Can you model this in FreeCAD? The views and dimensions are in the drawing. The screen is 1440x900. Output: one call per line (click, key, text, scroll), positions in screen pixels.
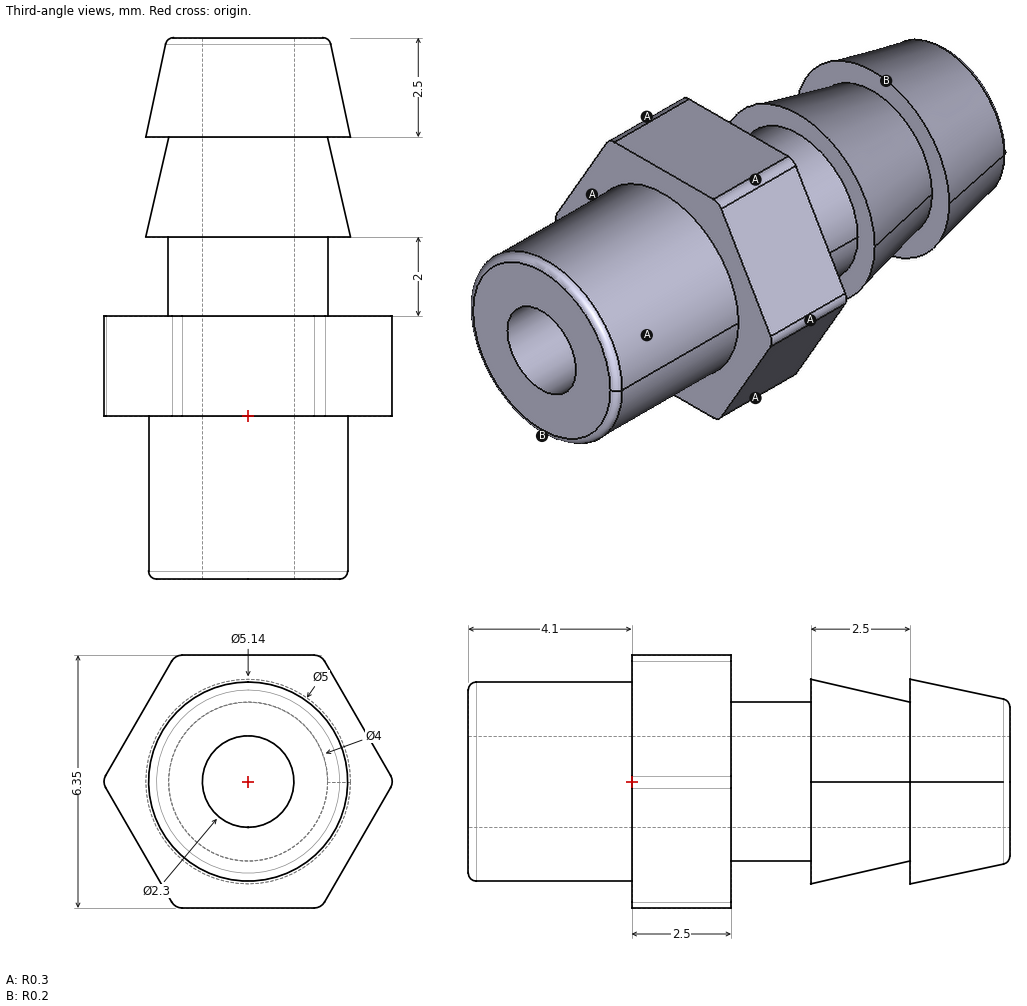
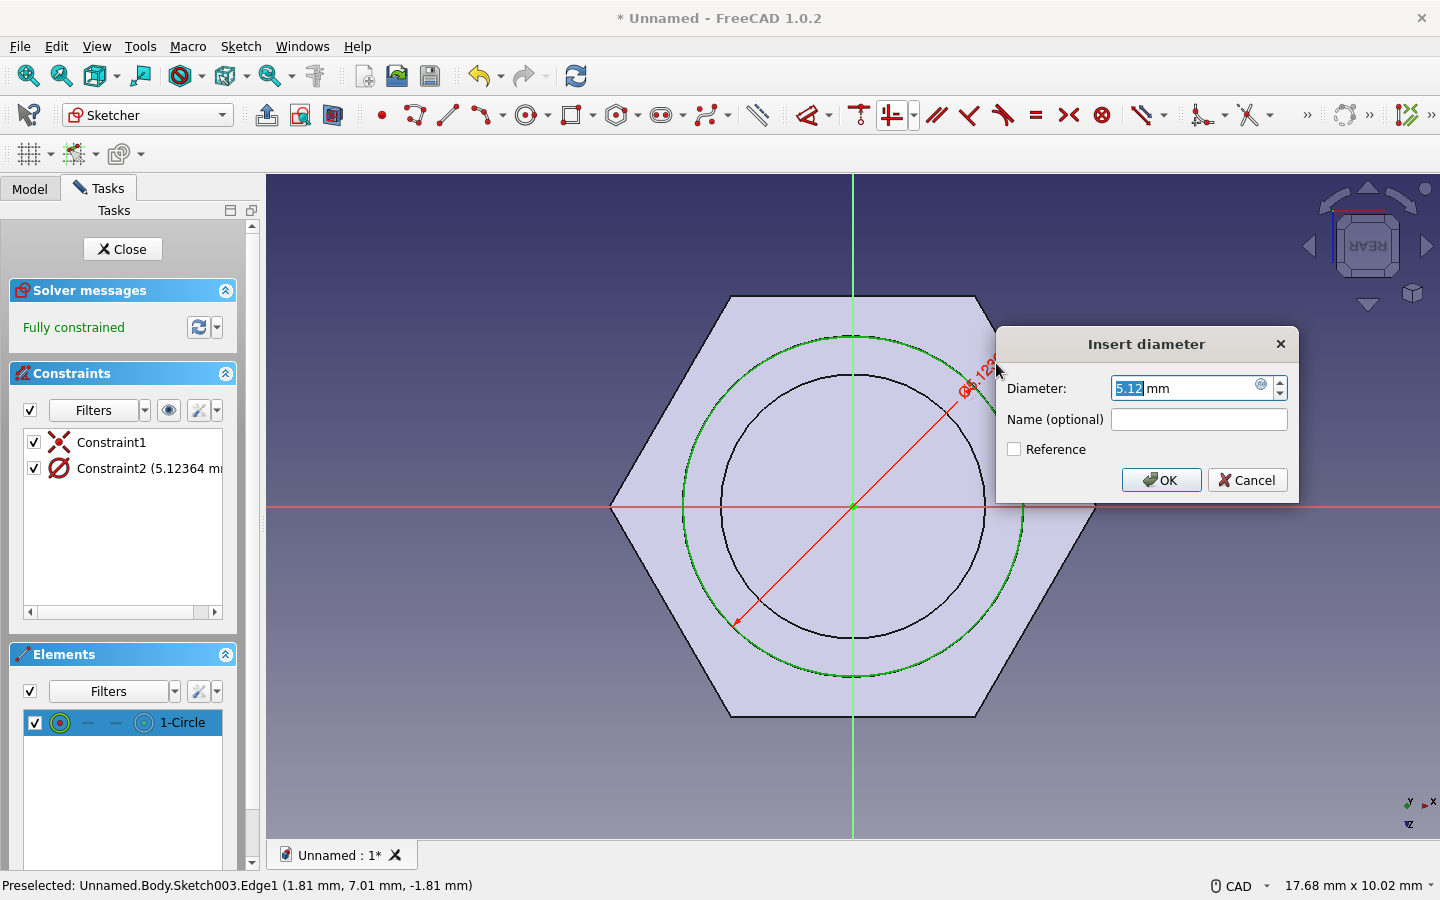
text(5.14)
key(Return)
key(Escape)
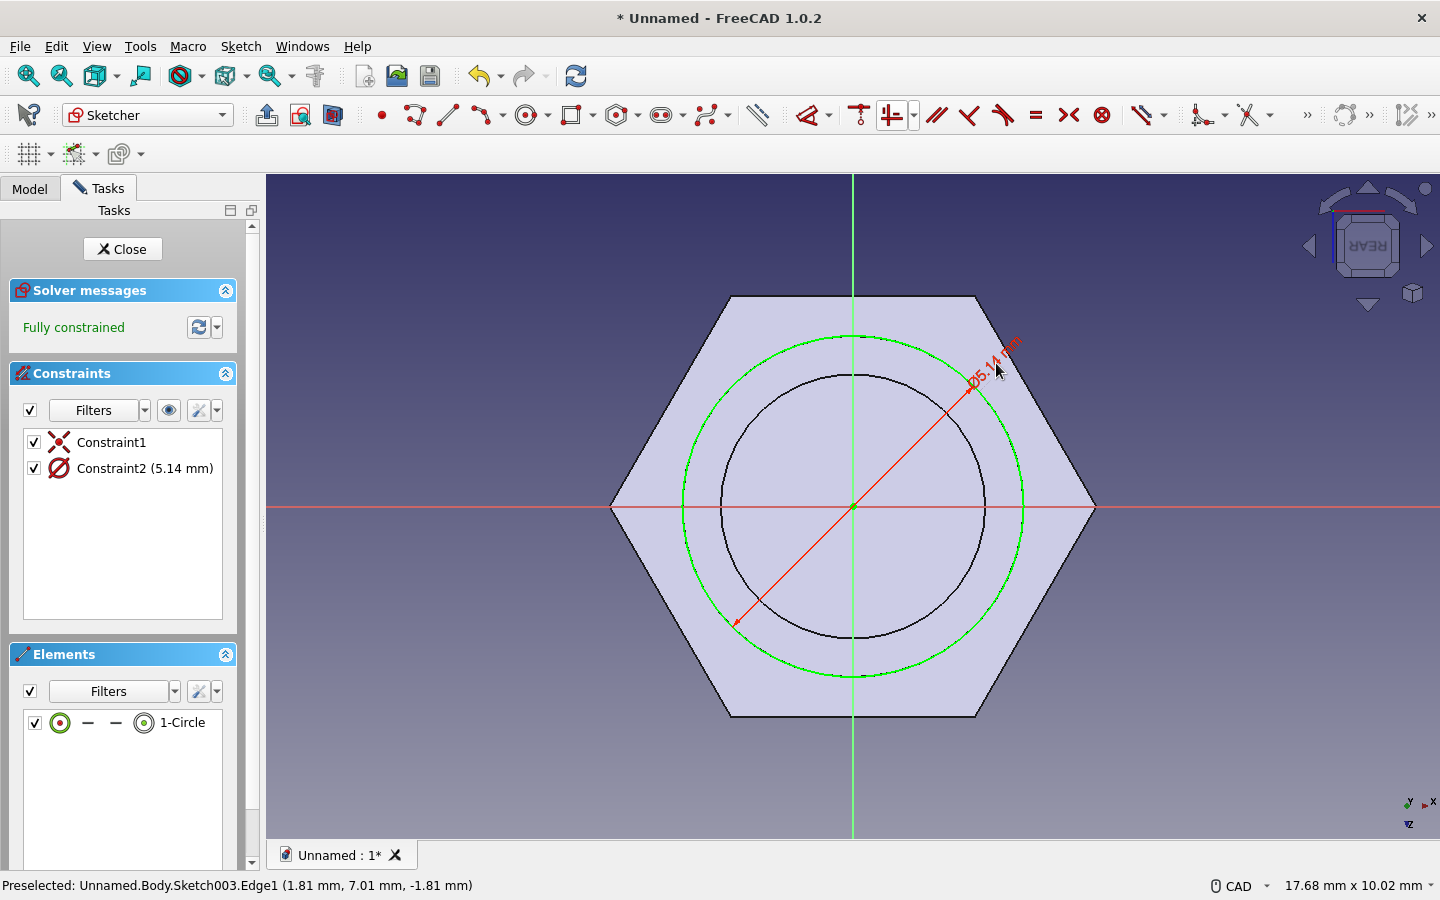
click(123, 249)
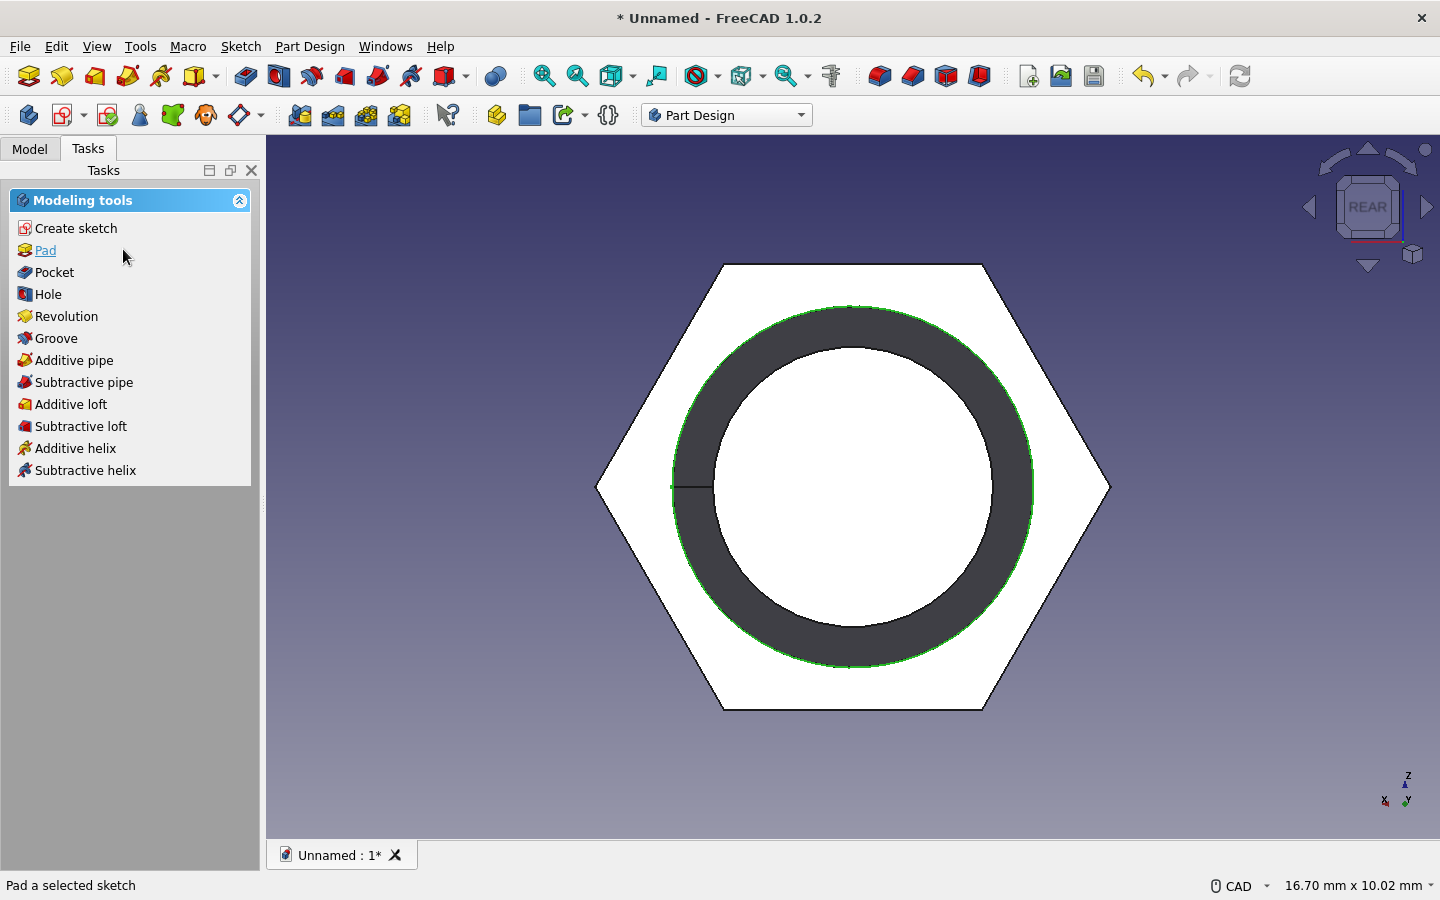
click(29, 76)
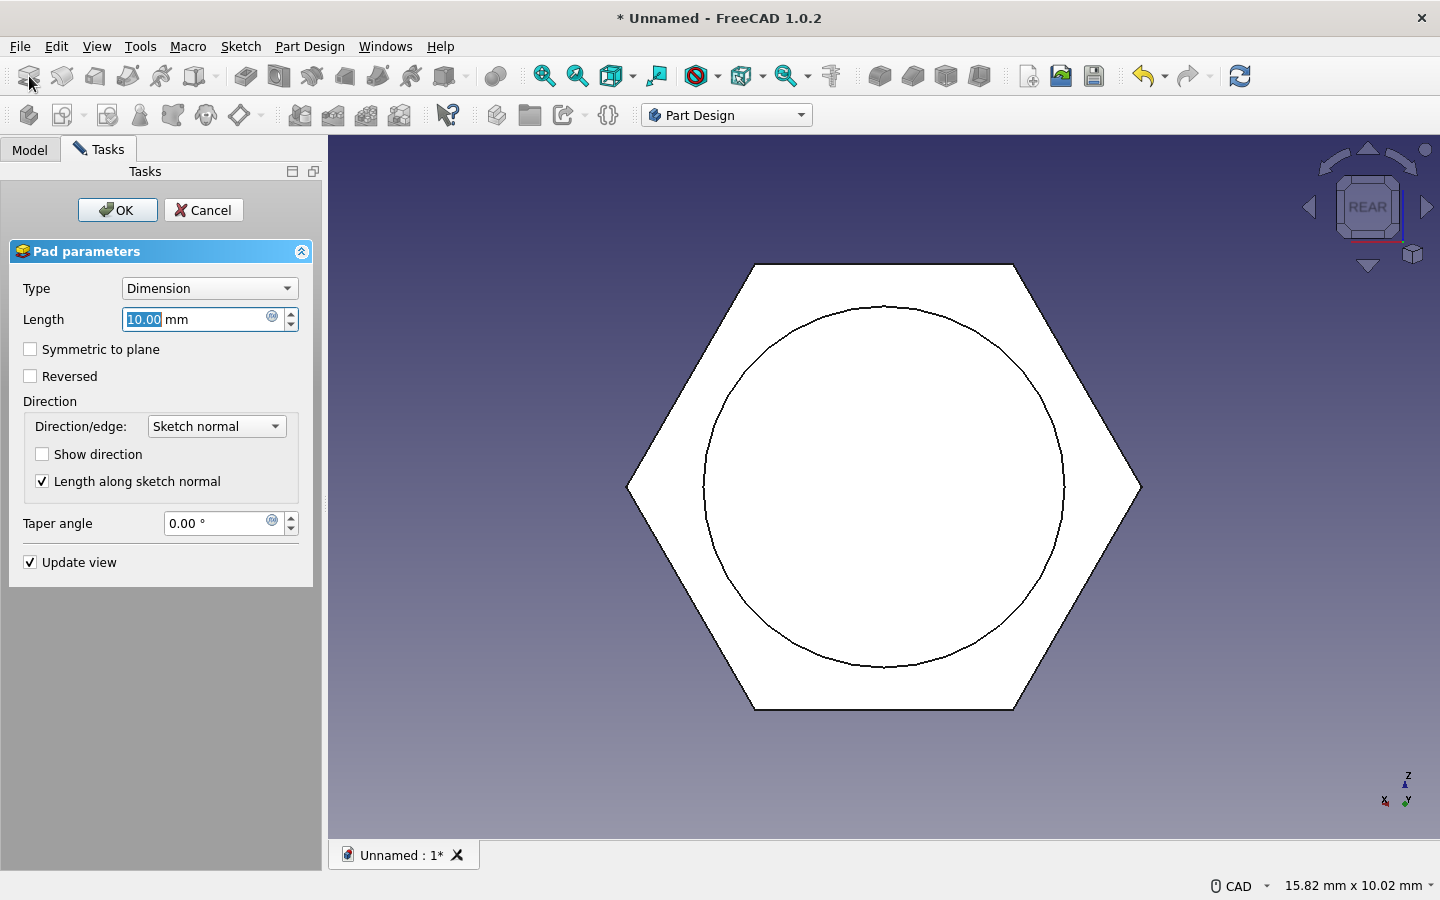
text(2.5)
key(Tab)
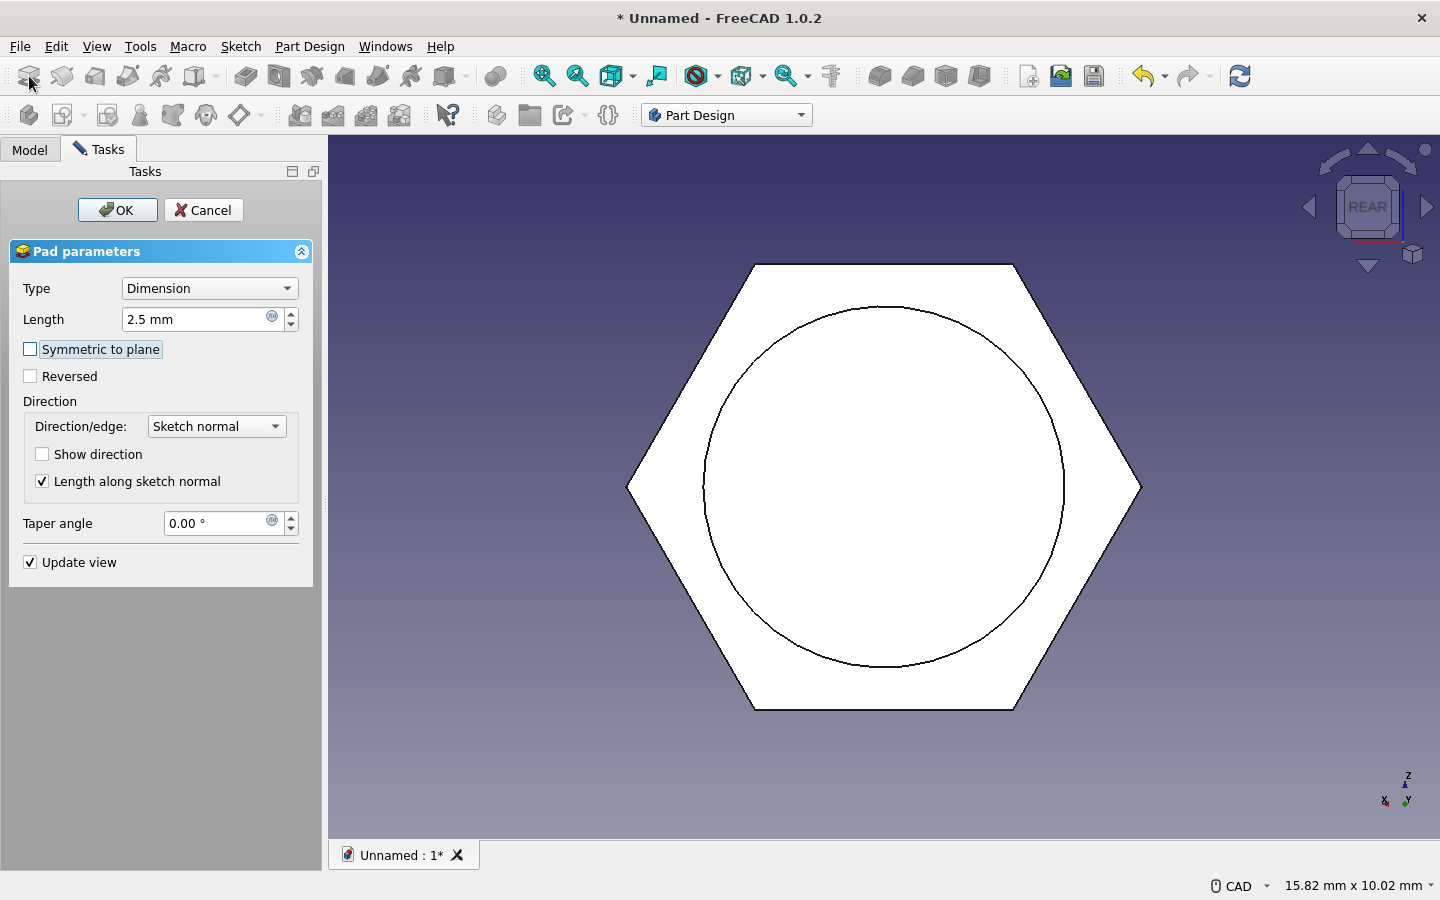
triple_click(224, 524)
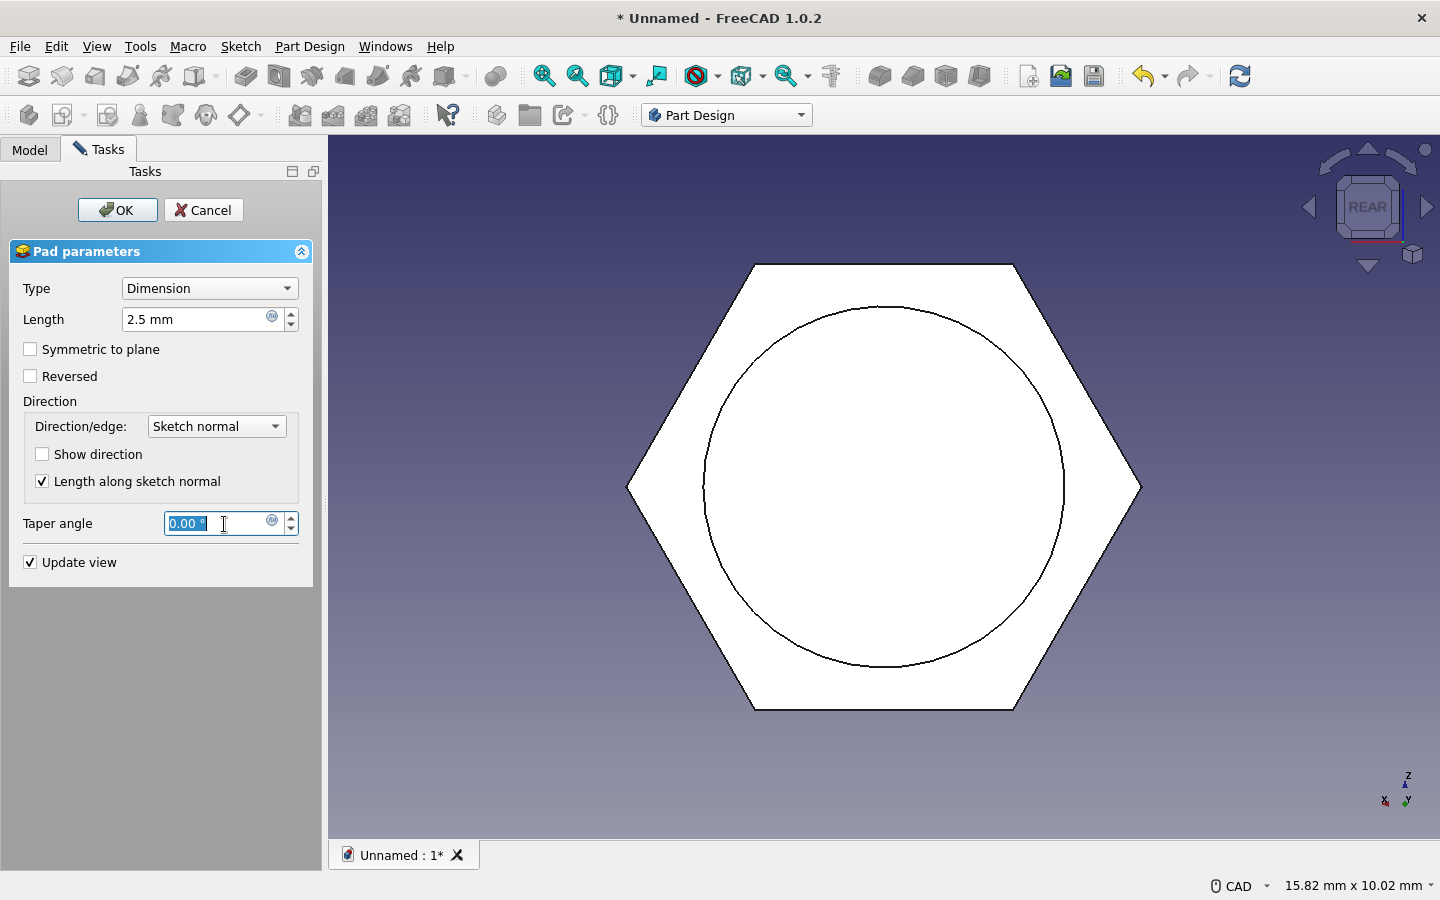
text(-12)
key(Tab)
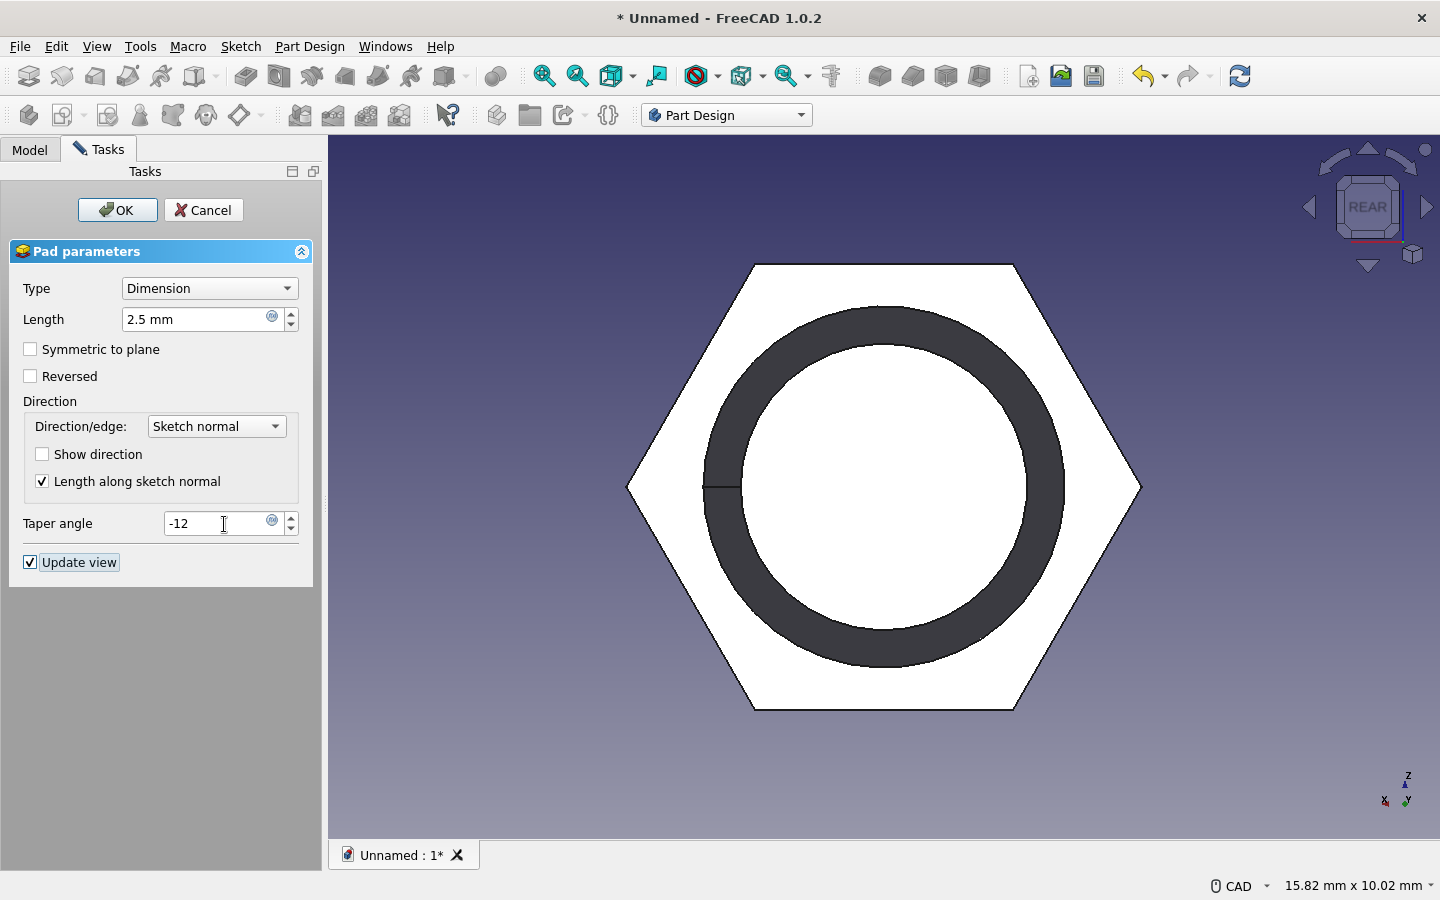
click(118, 210)